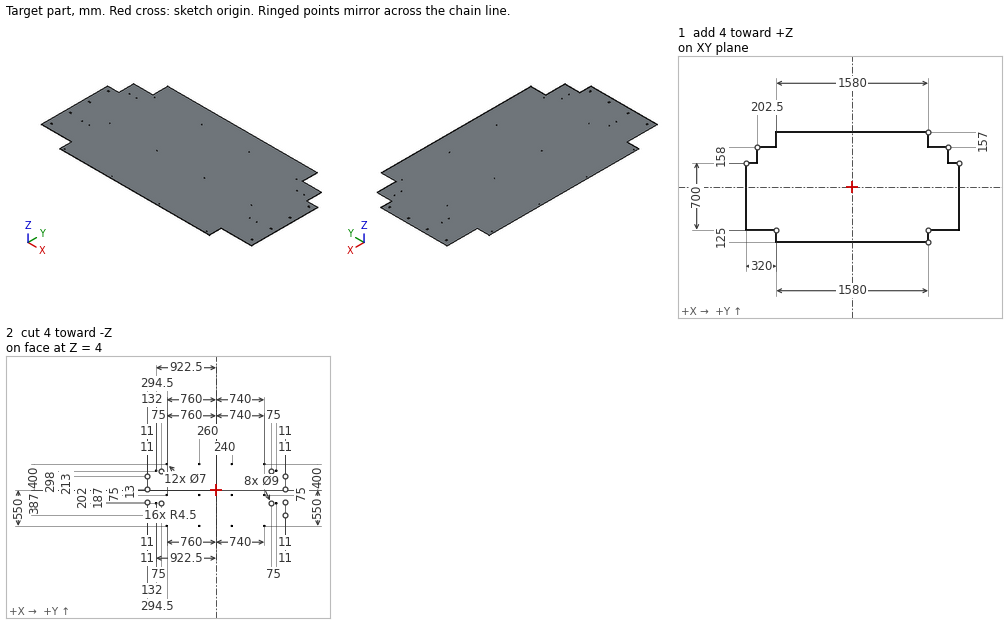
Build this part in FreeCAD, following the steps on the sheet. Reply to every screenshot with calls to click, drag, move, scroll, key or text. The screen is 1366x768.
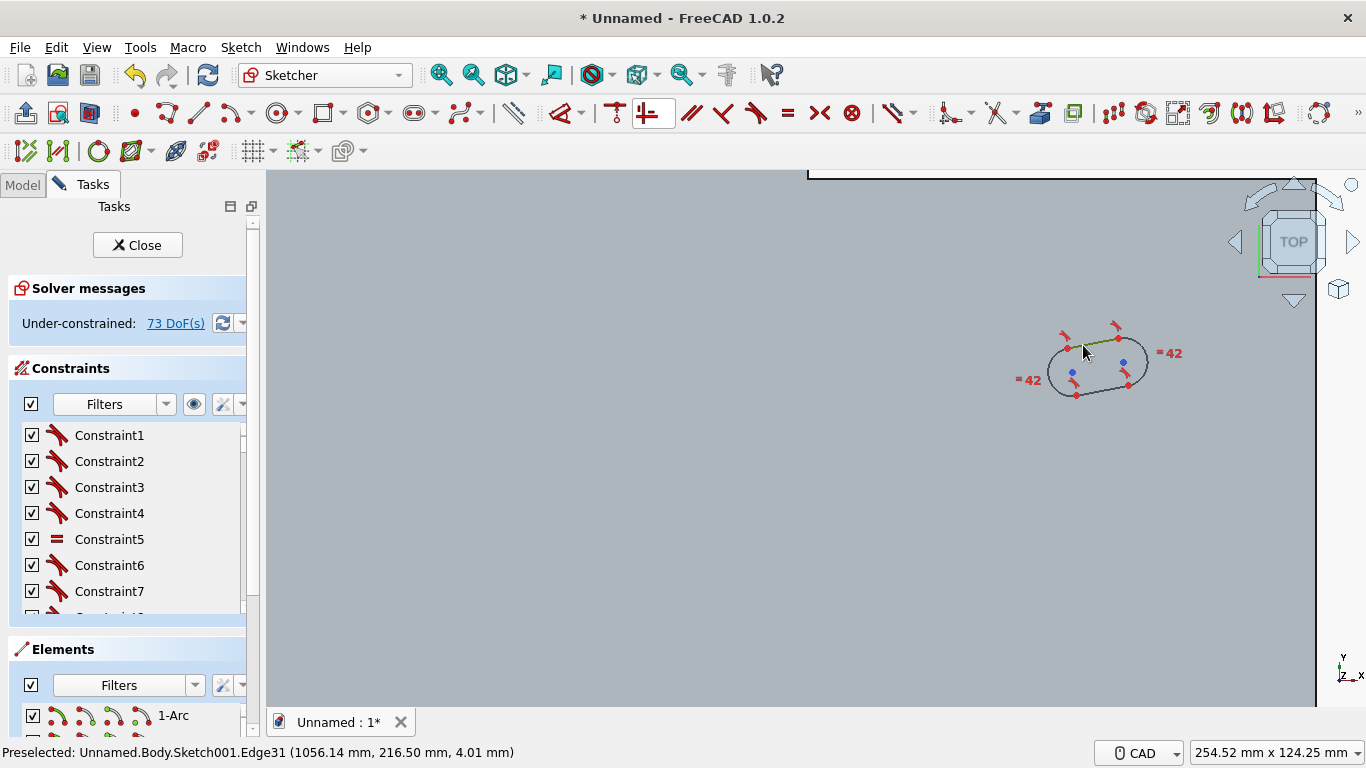
key(h)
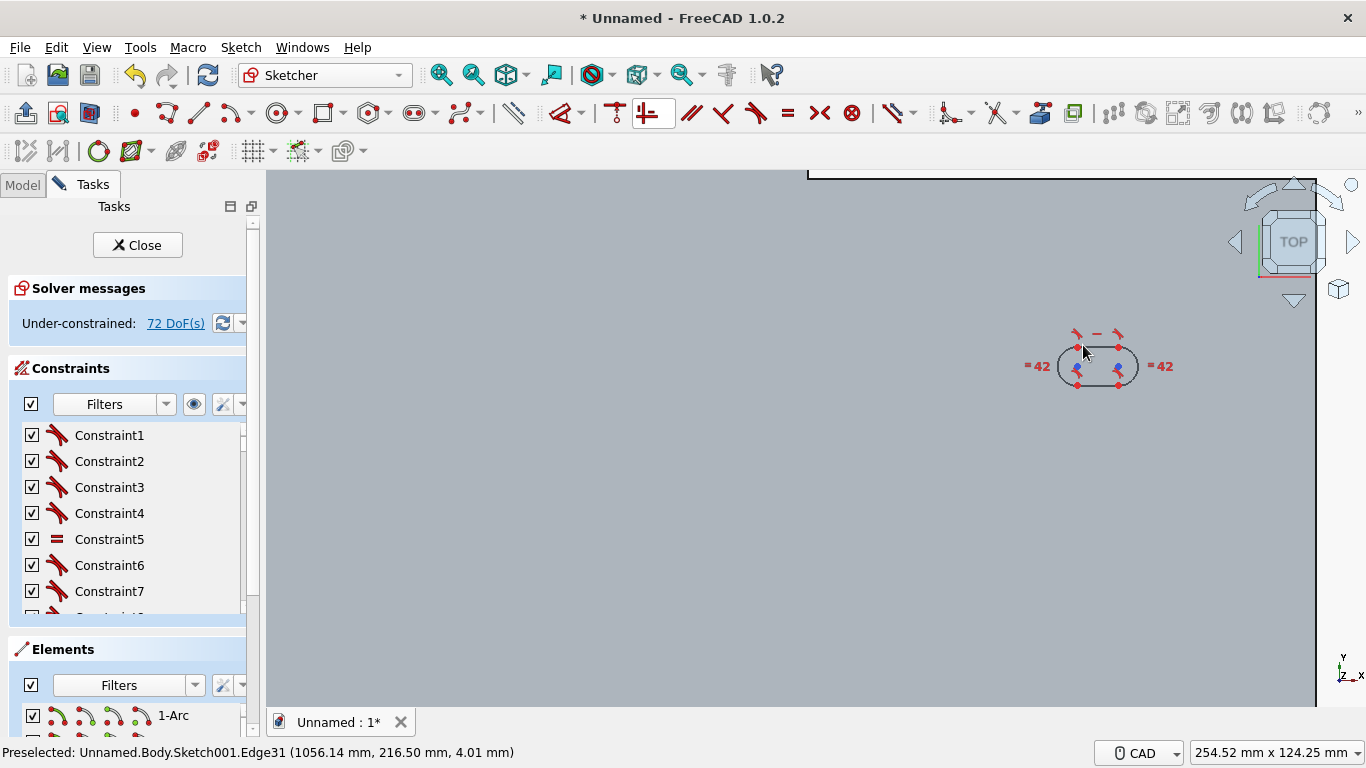
scroll(1087, 345, down, 13)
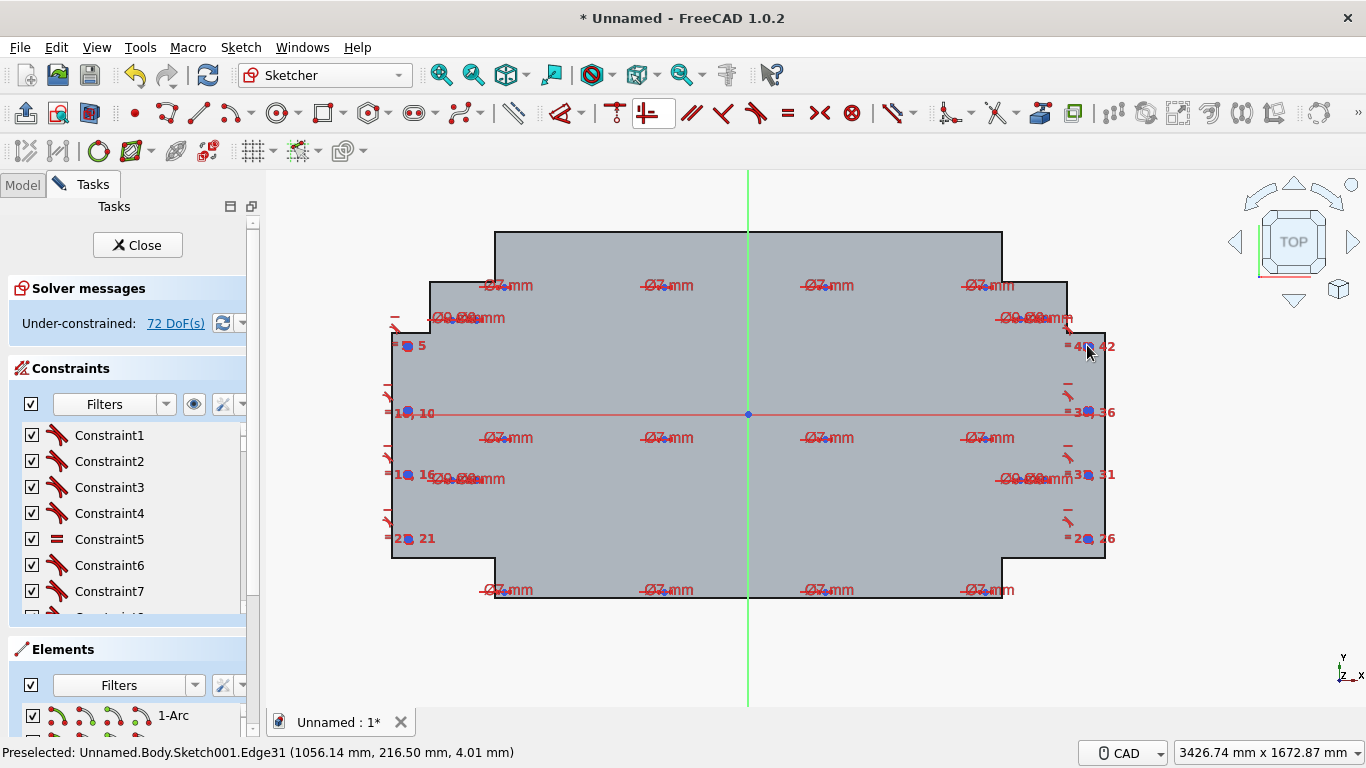
scroll(405, 346, up, 11)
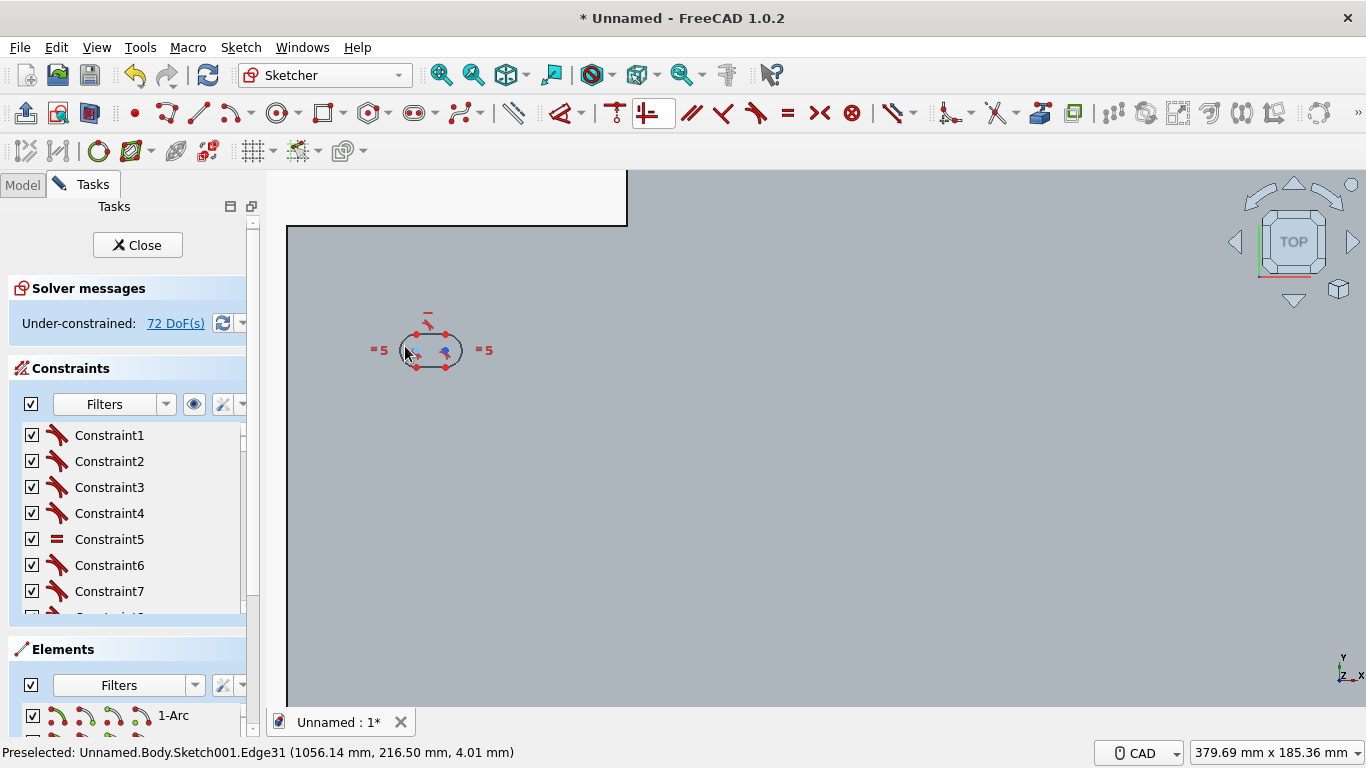
click(403, 341)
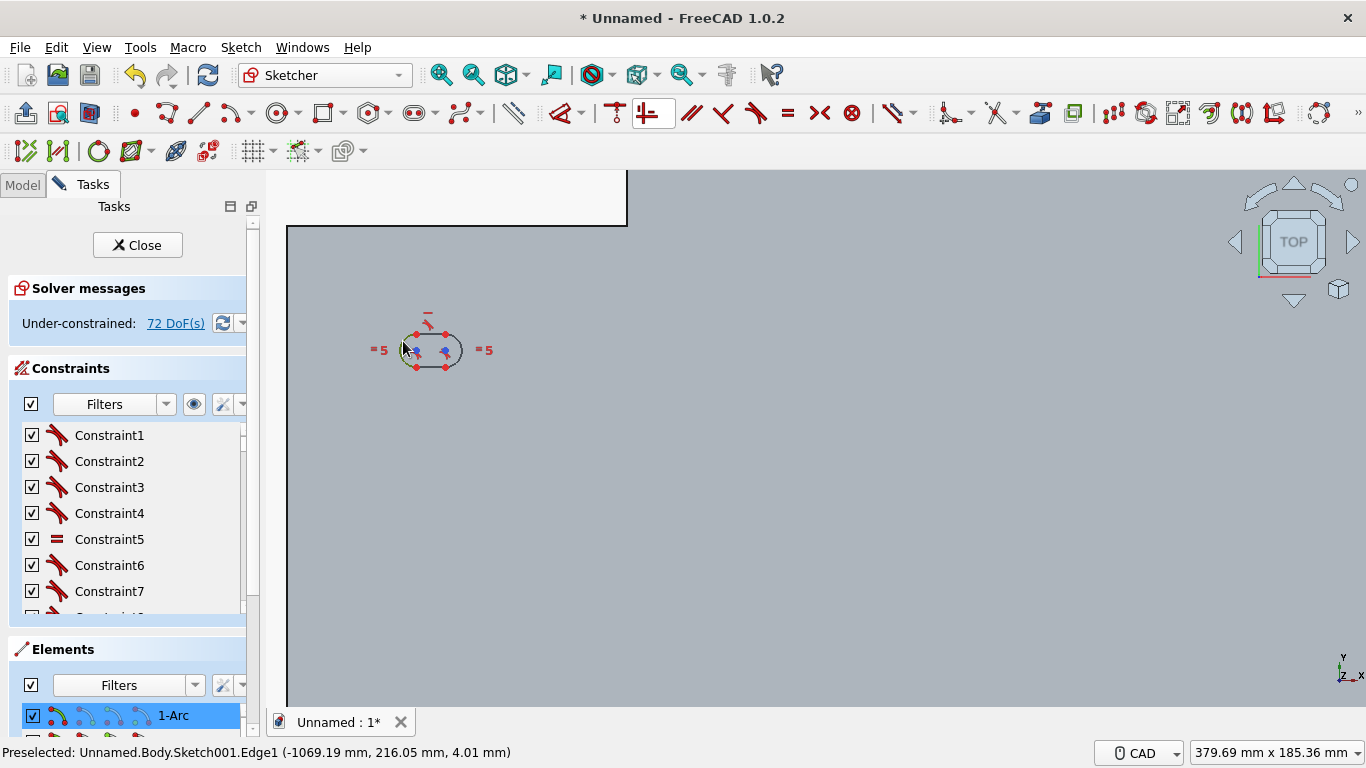
scroll(404, 346, down, 11)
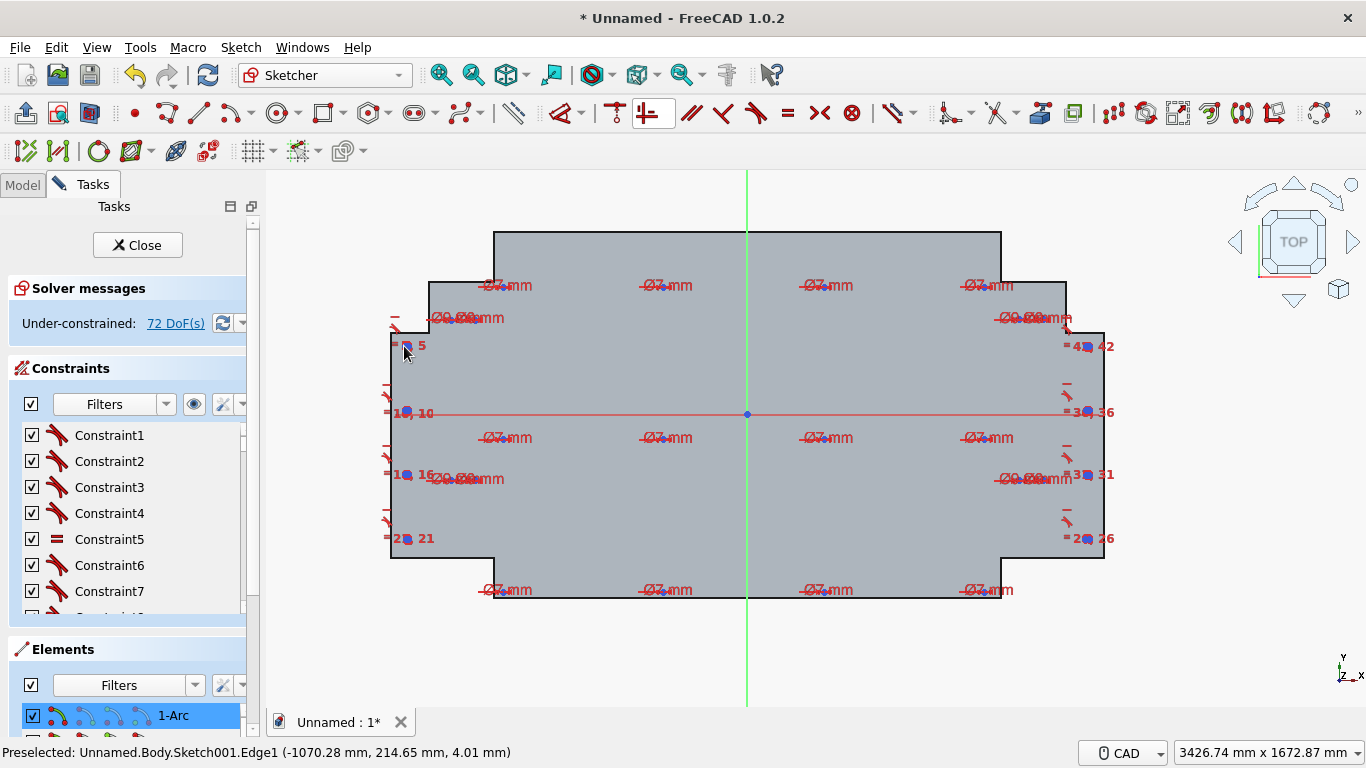
scroll(404, 410, up, 12)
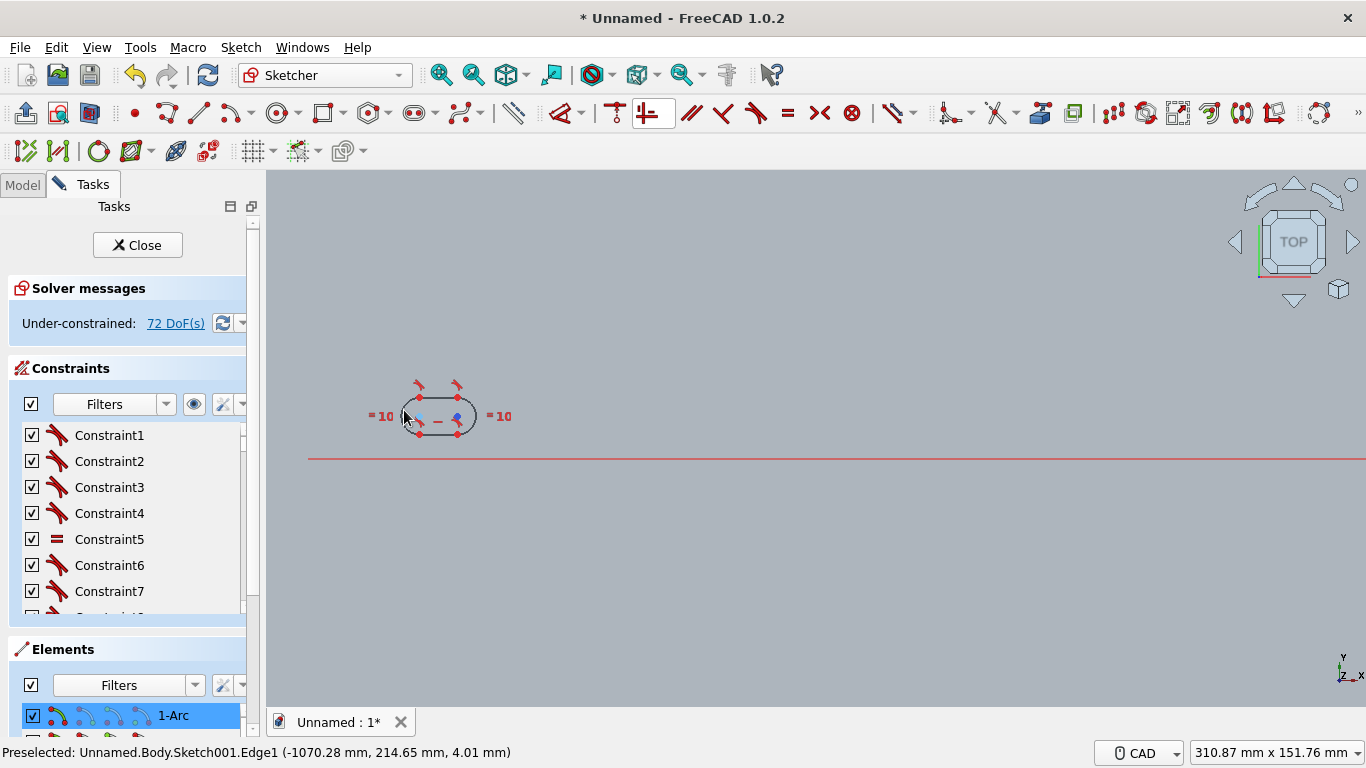
click(405, 406)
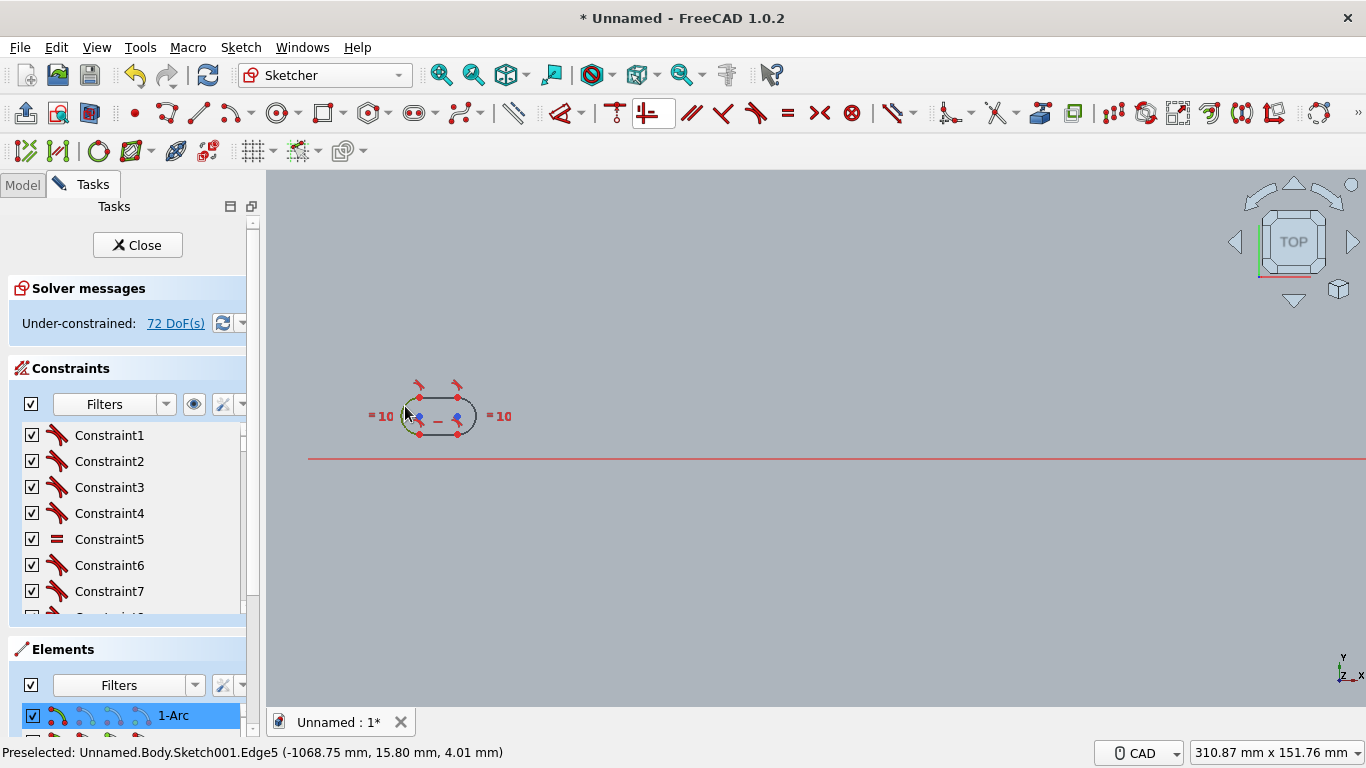
scroll(404, 410, down, 12)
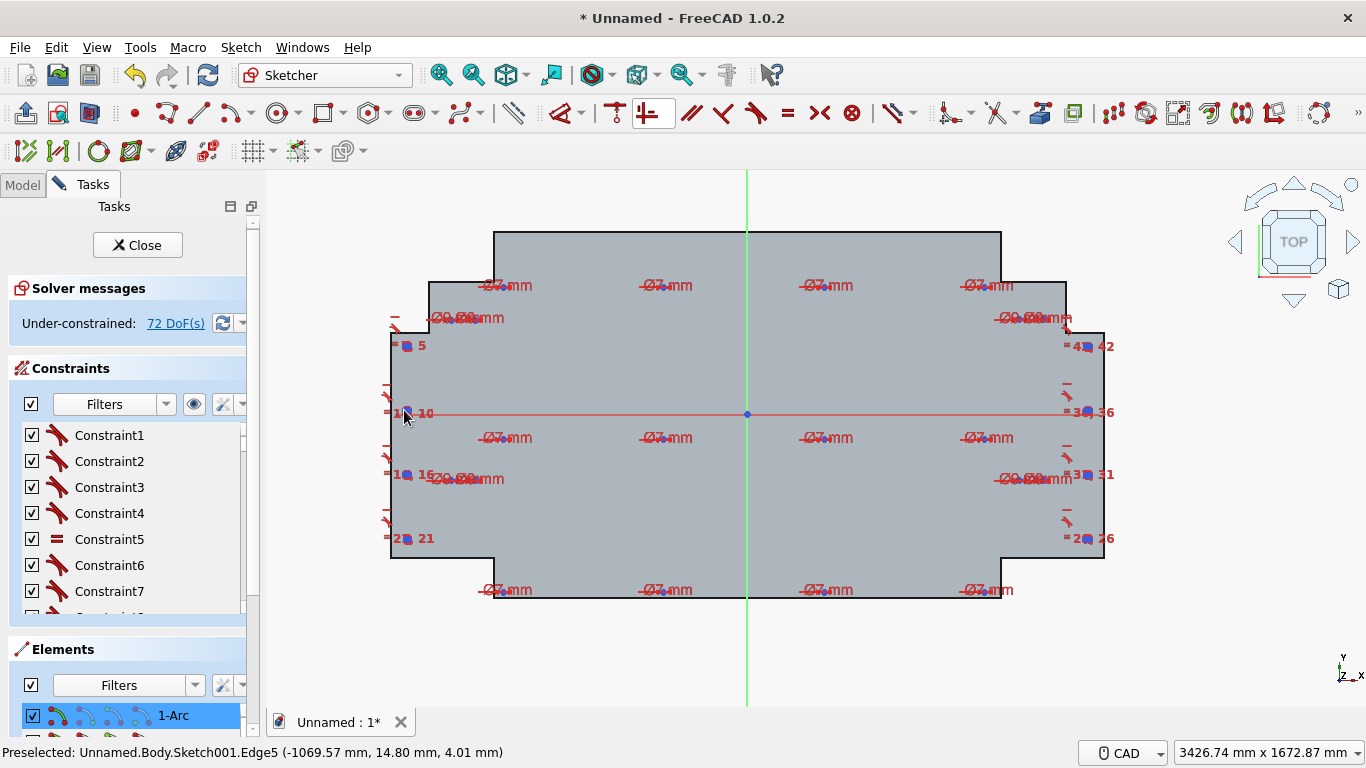
scroll(405, 474, up, 13)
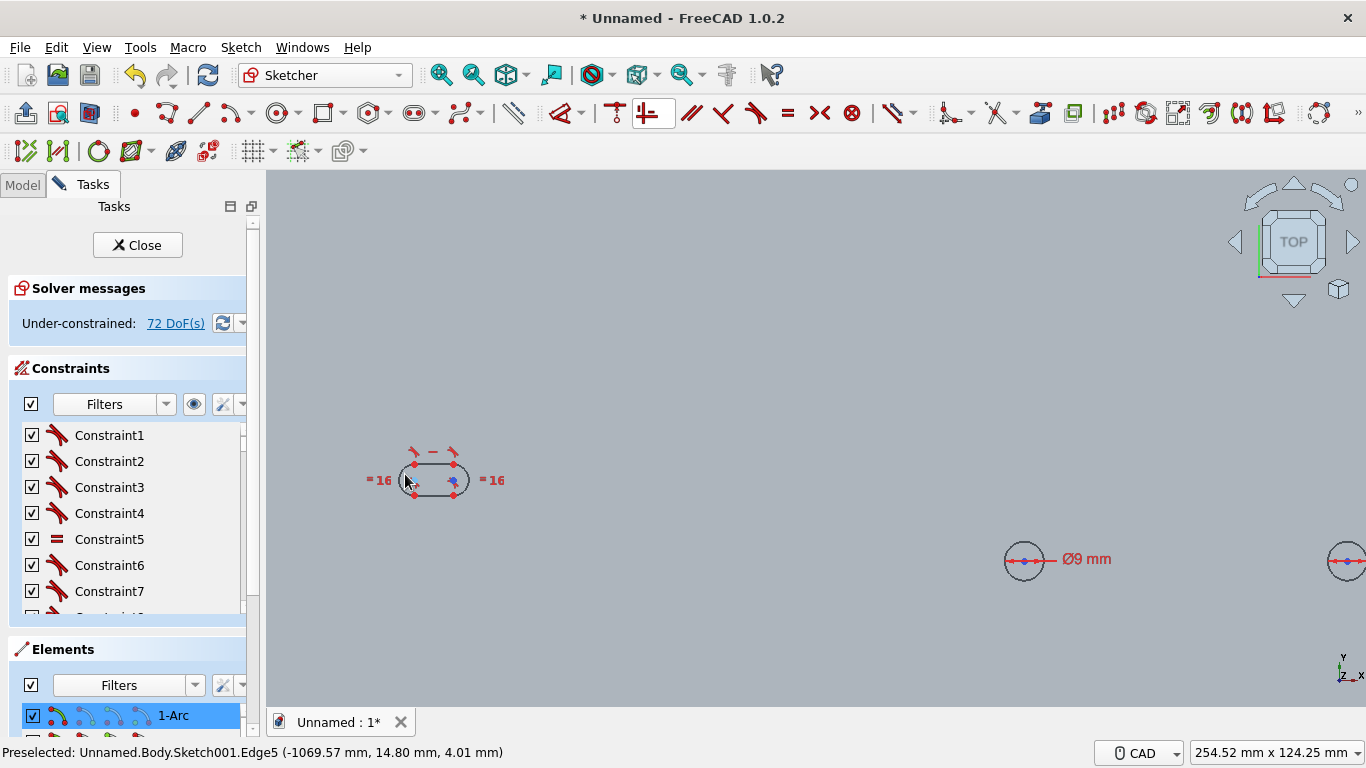
click(402, 471)